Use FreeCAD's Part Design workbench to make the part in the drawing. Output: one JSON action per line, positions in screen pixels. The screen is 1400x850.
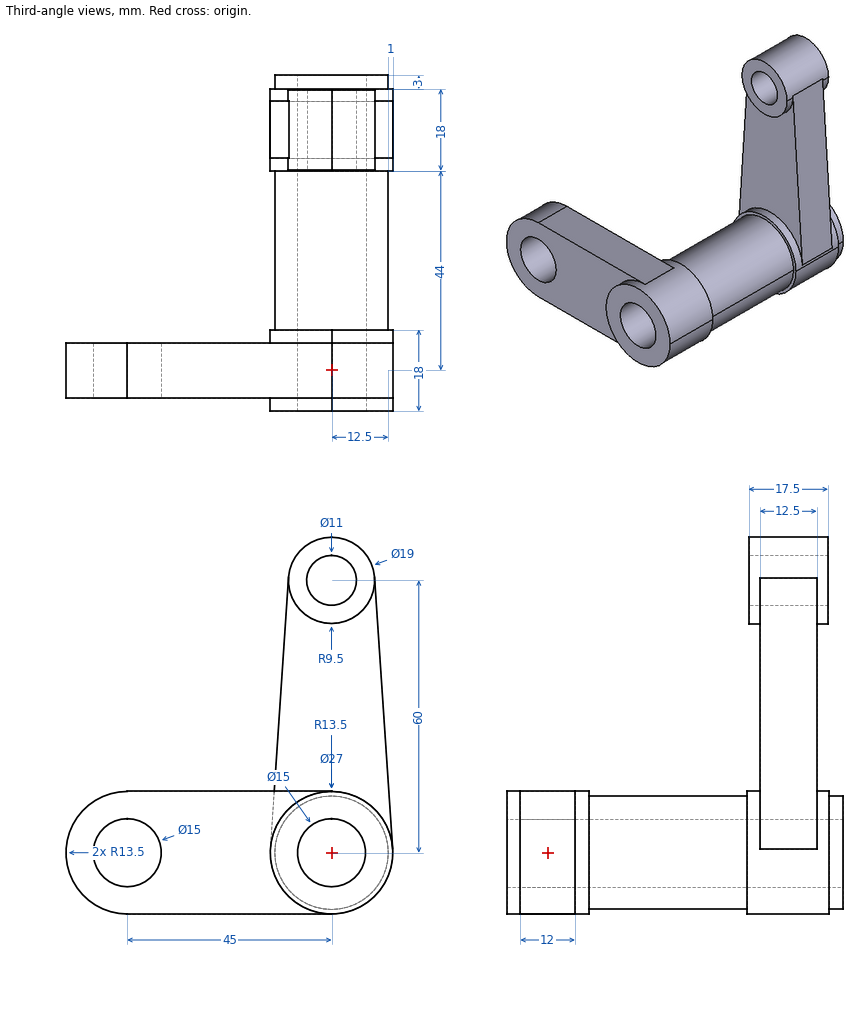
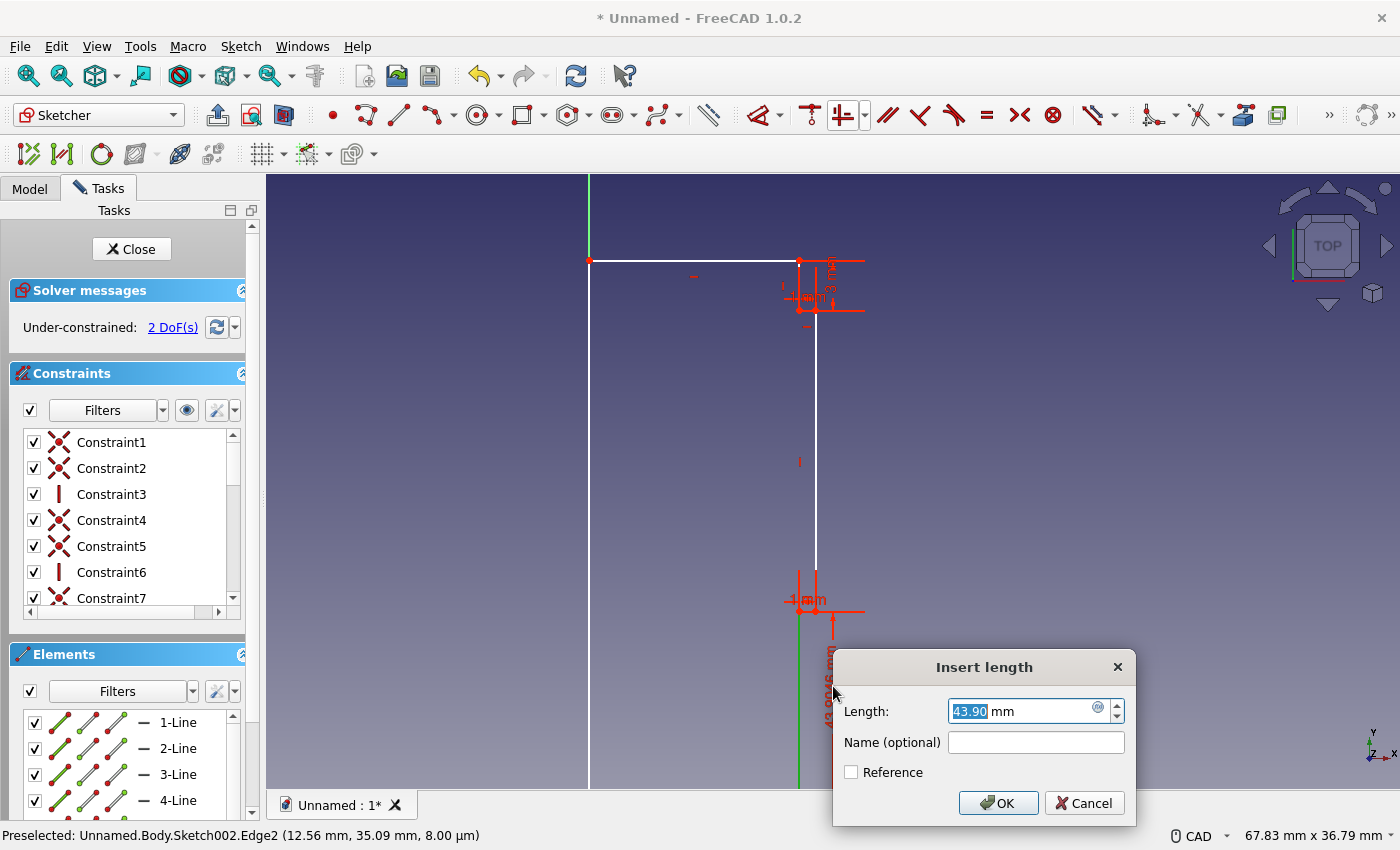
{"action": "type", "text": "44"}
{"action": "key", "text": "Return"}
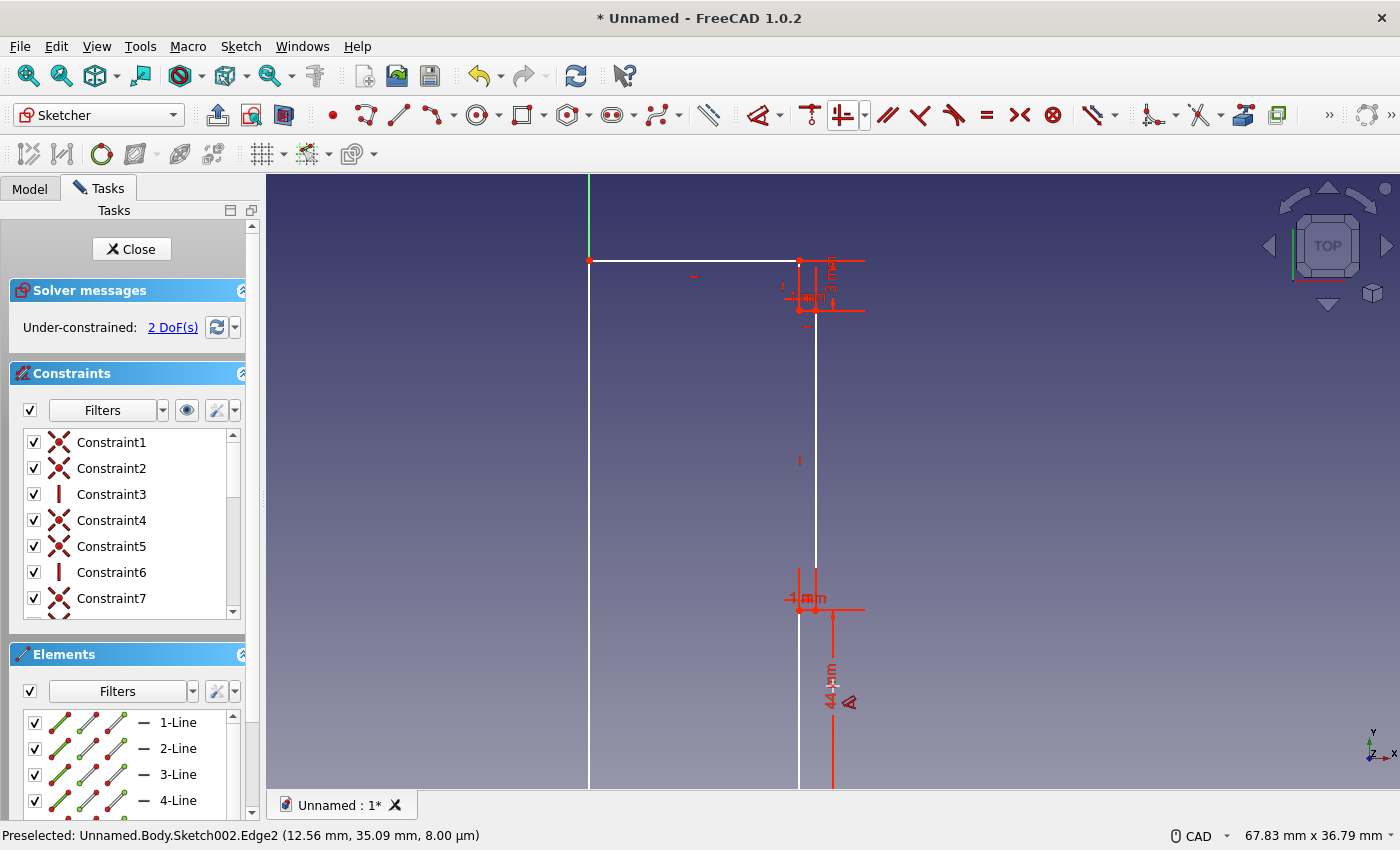
{"action": "left_click", "coordinate": [816, 520]}
{"action": "left_click", "coordinate": [850, 461]}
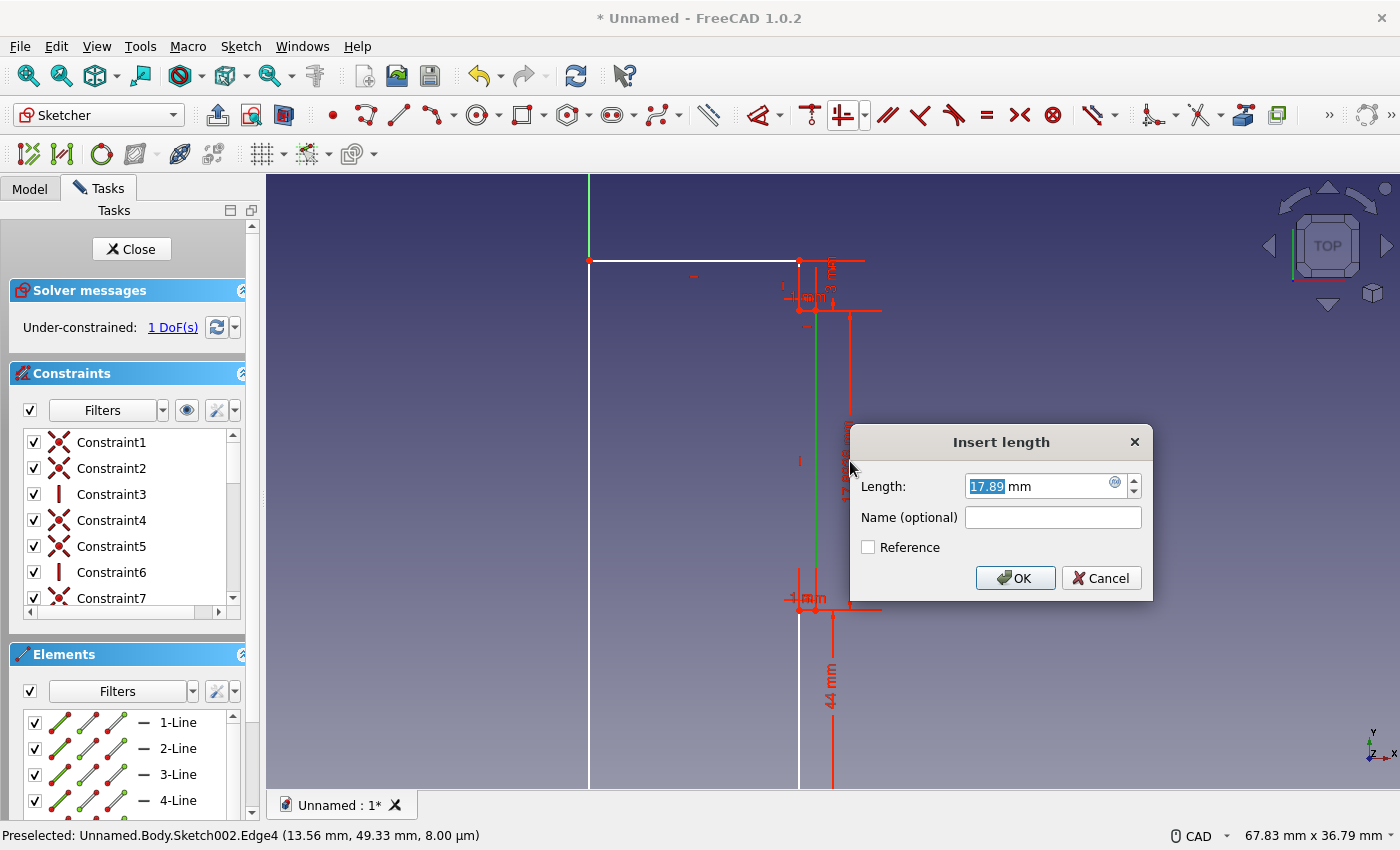
{"action": "type", "text": "18"}
{"action": "key", "text": "Return"}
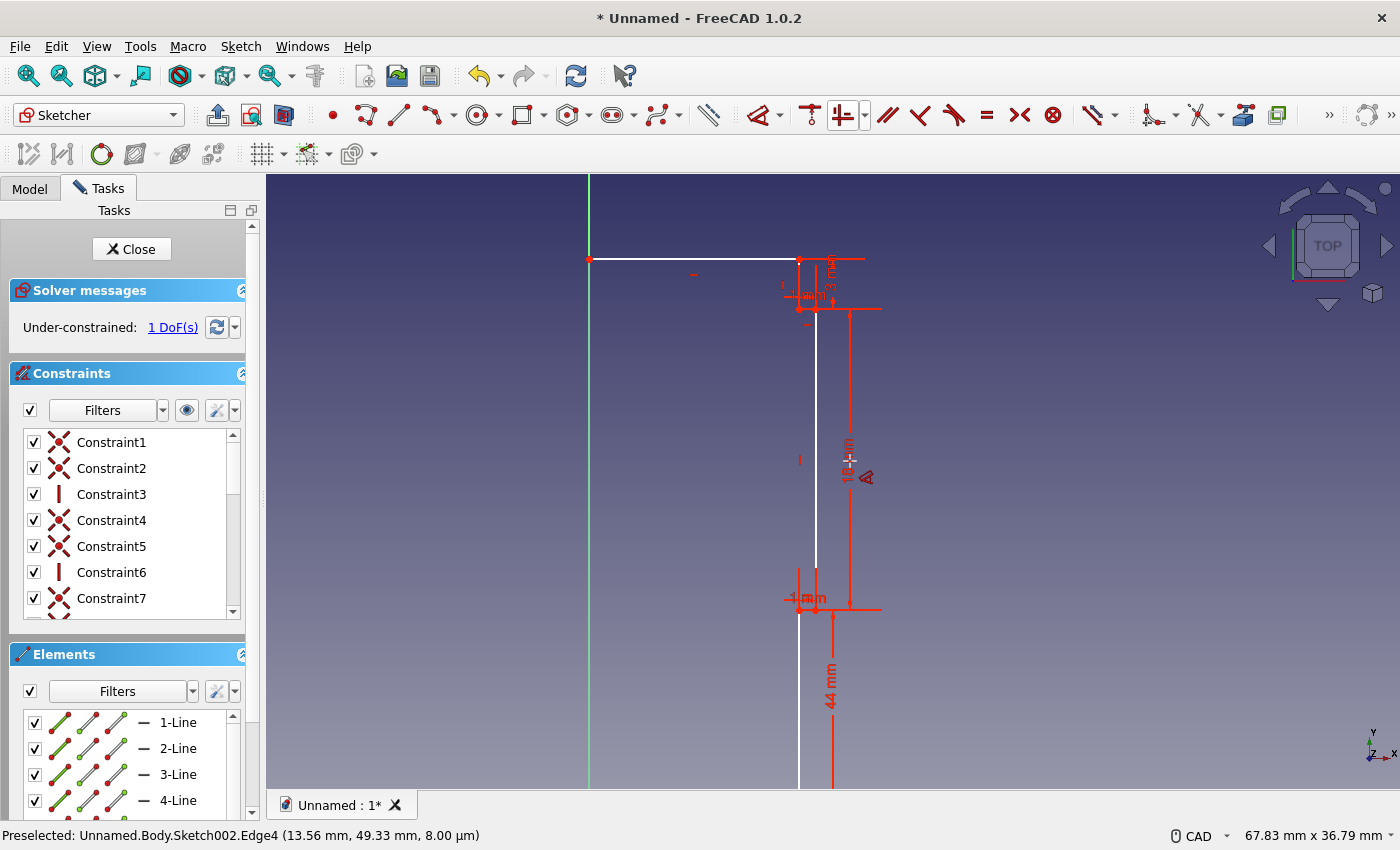
{"action": "scroll", "coordinate": [801, 295], "scroll_direction": "down", "scroll_amount": 5}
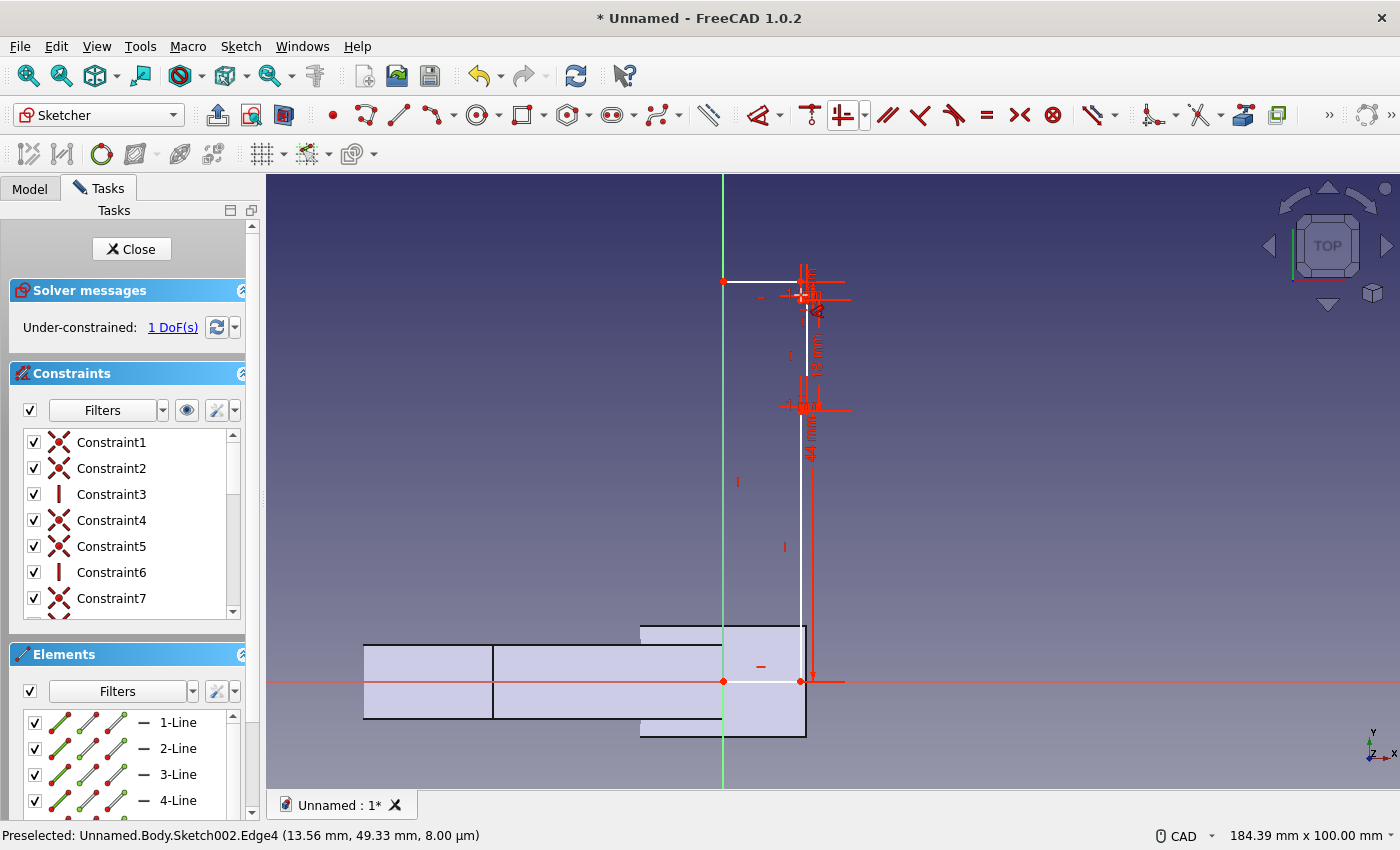
{"action": "left_click", "coordinate": [747, 682]}
{"action": "left_click", "coordinate": [762, 716]}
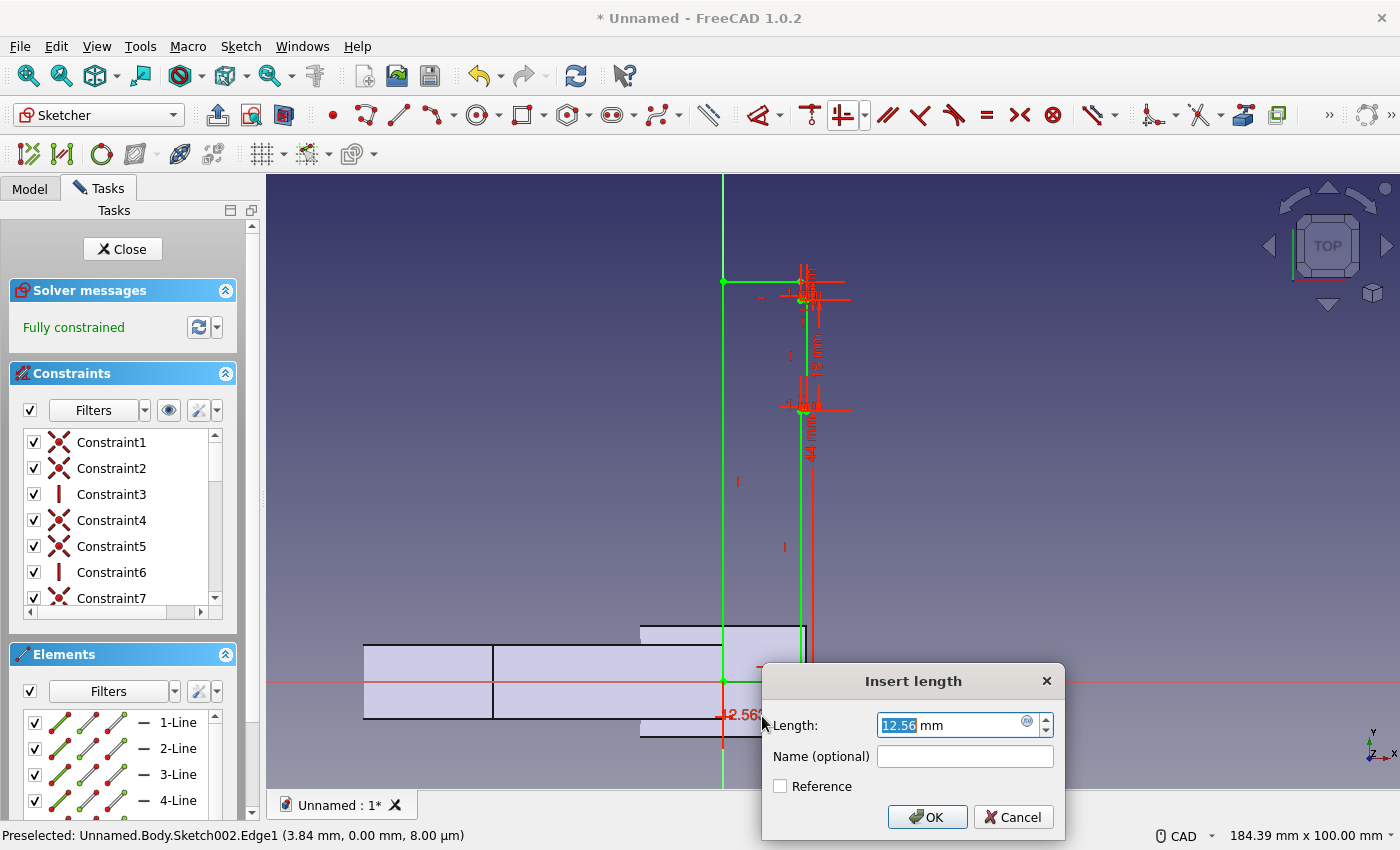
{"action": "type", "text": "12.5"}
{"action": "key", "text": "Return"}
{"action": "key", "text": "Escape"}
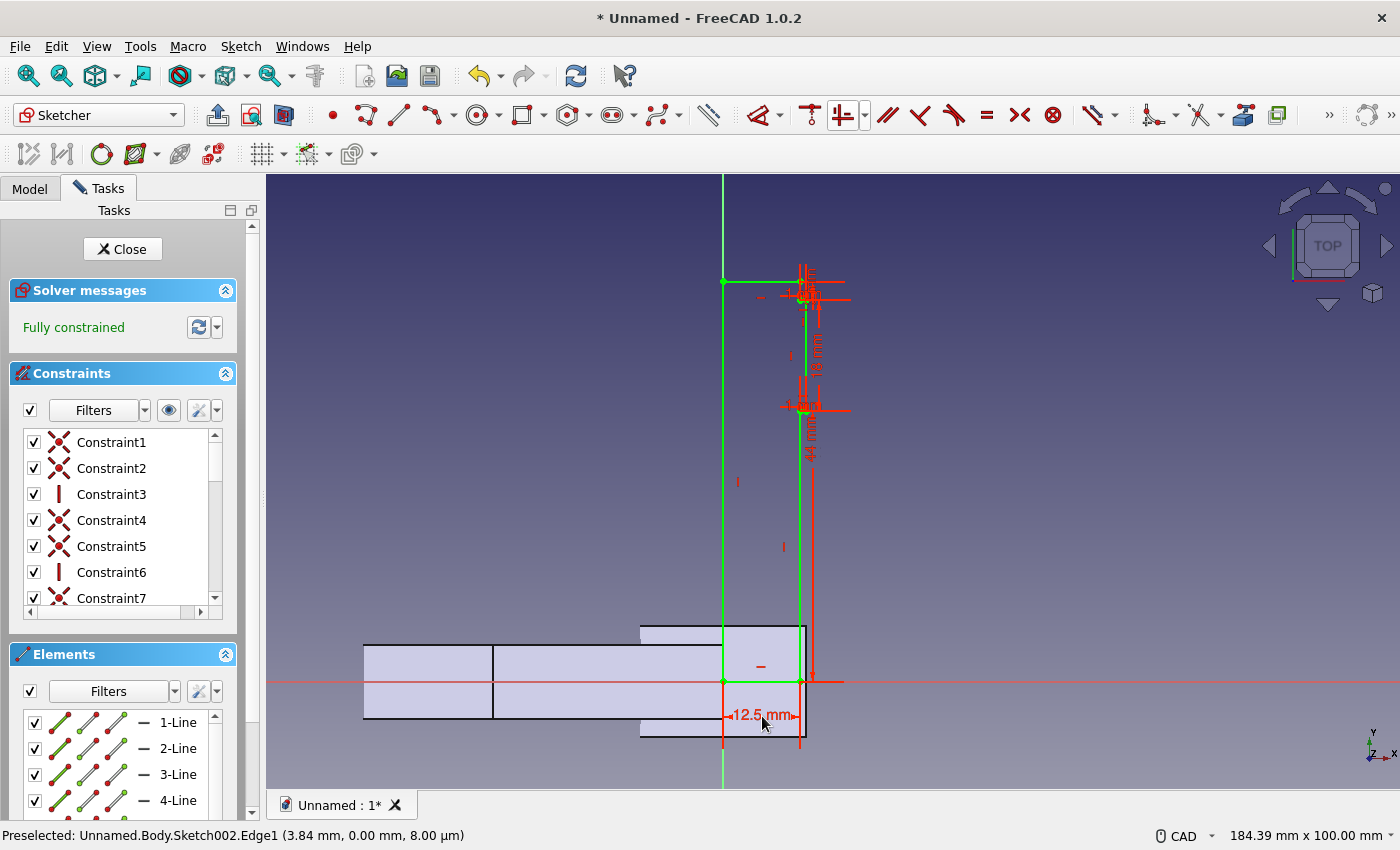
{"action": "left_click", "coordinate": [123, 249]}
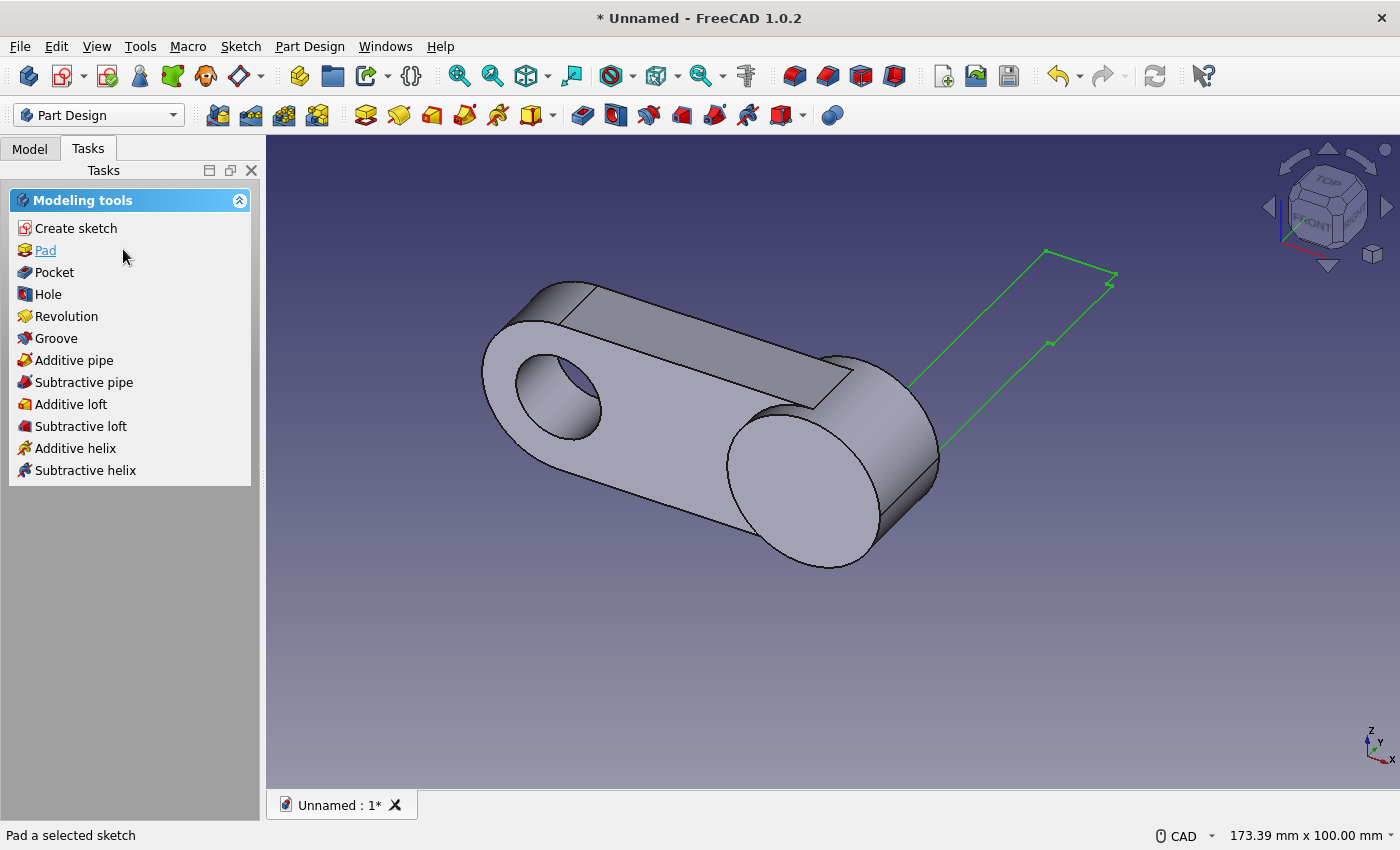
{"action": "left_click", "coordinate": [399, 116]}